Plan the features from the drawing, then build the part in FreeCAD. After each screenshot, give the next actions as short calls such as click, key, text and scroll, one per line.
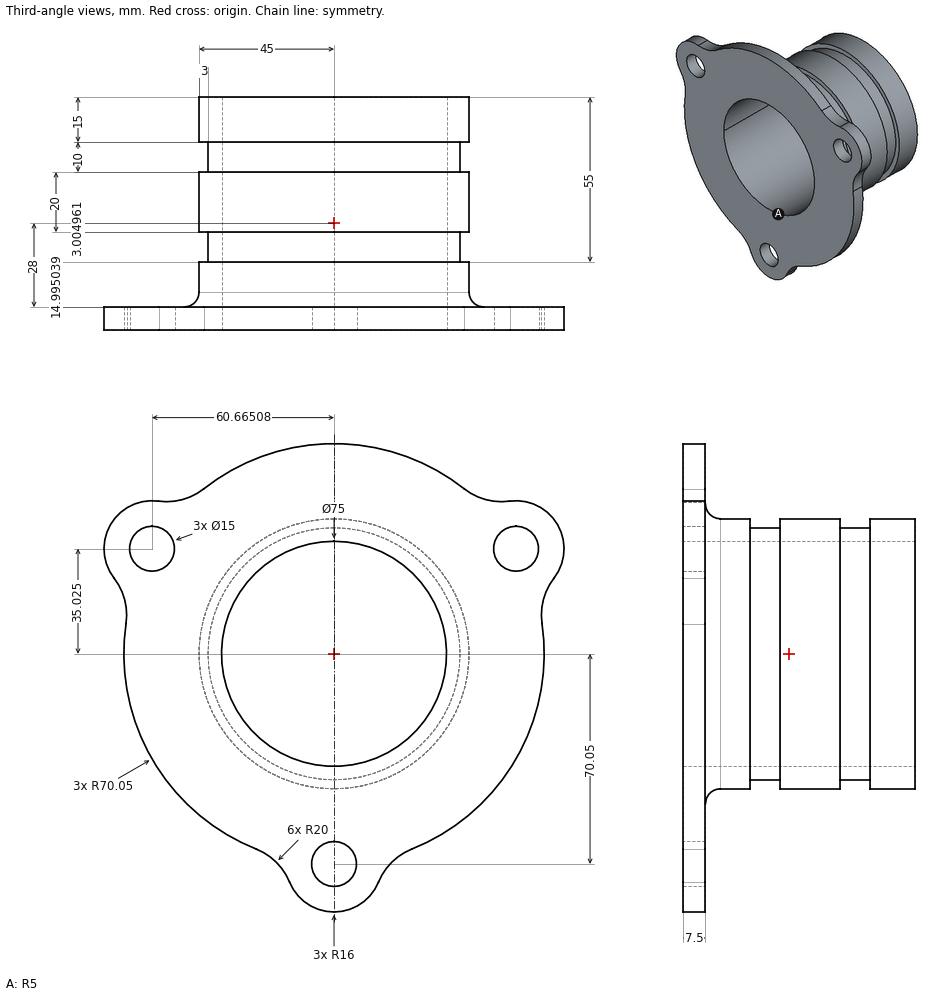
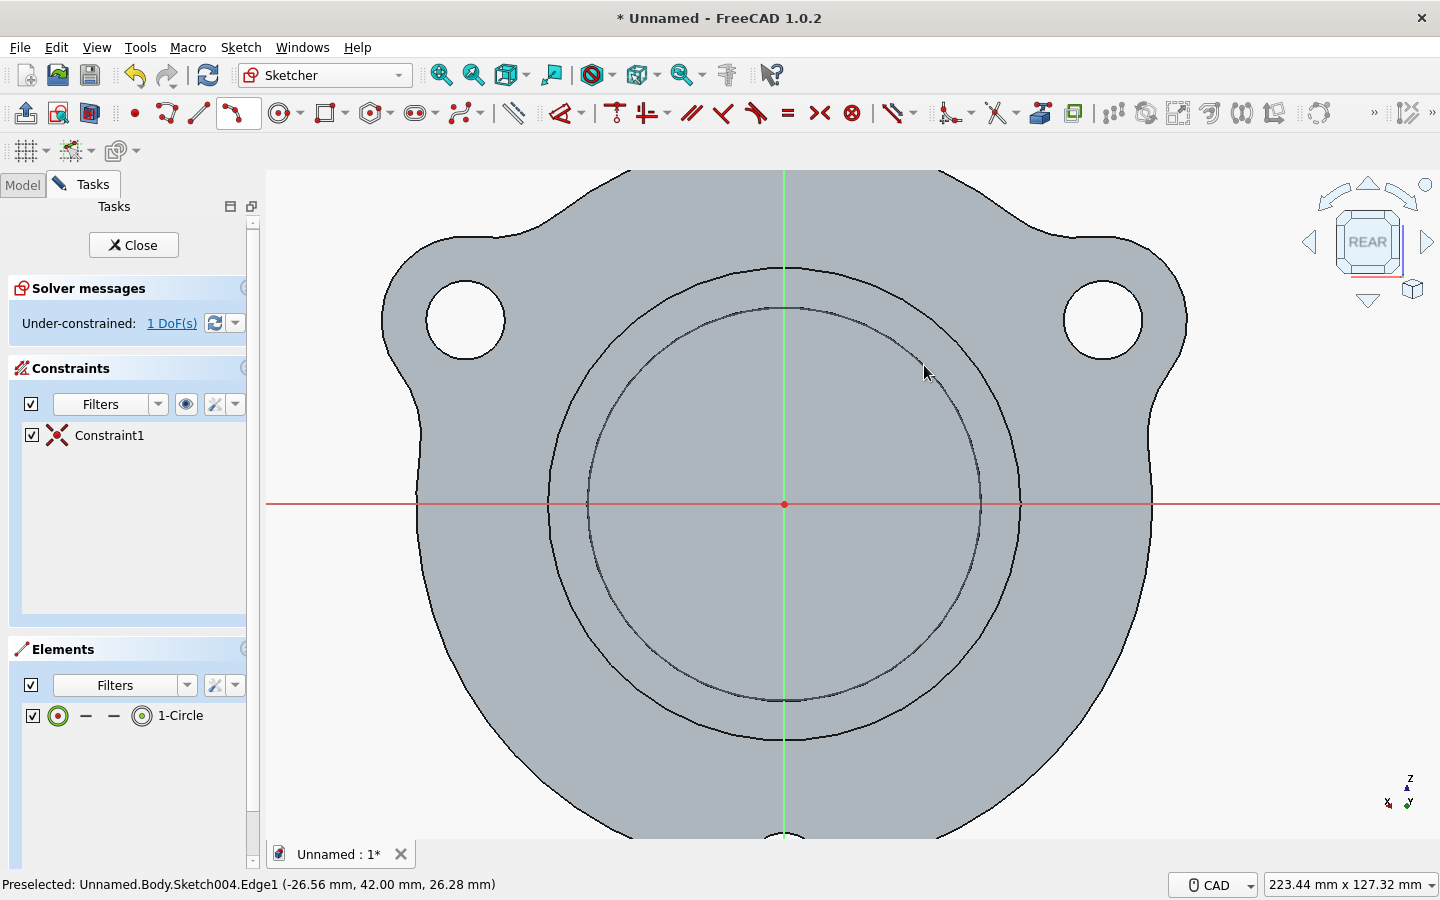
click(560, 114)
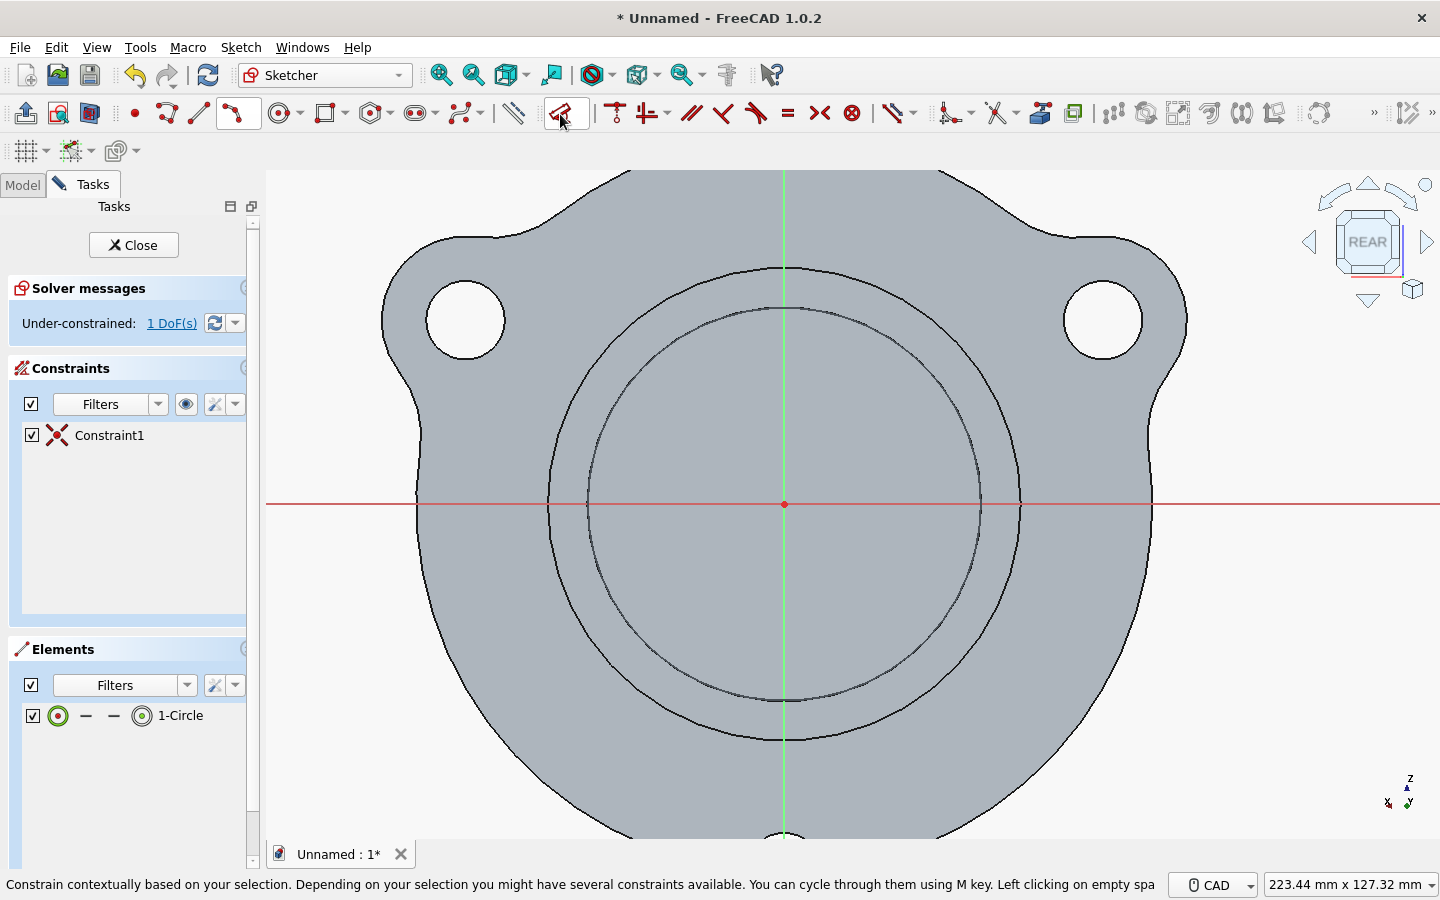
click(923, 365)
click(946, 342)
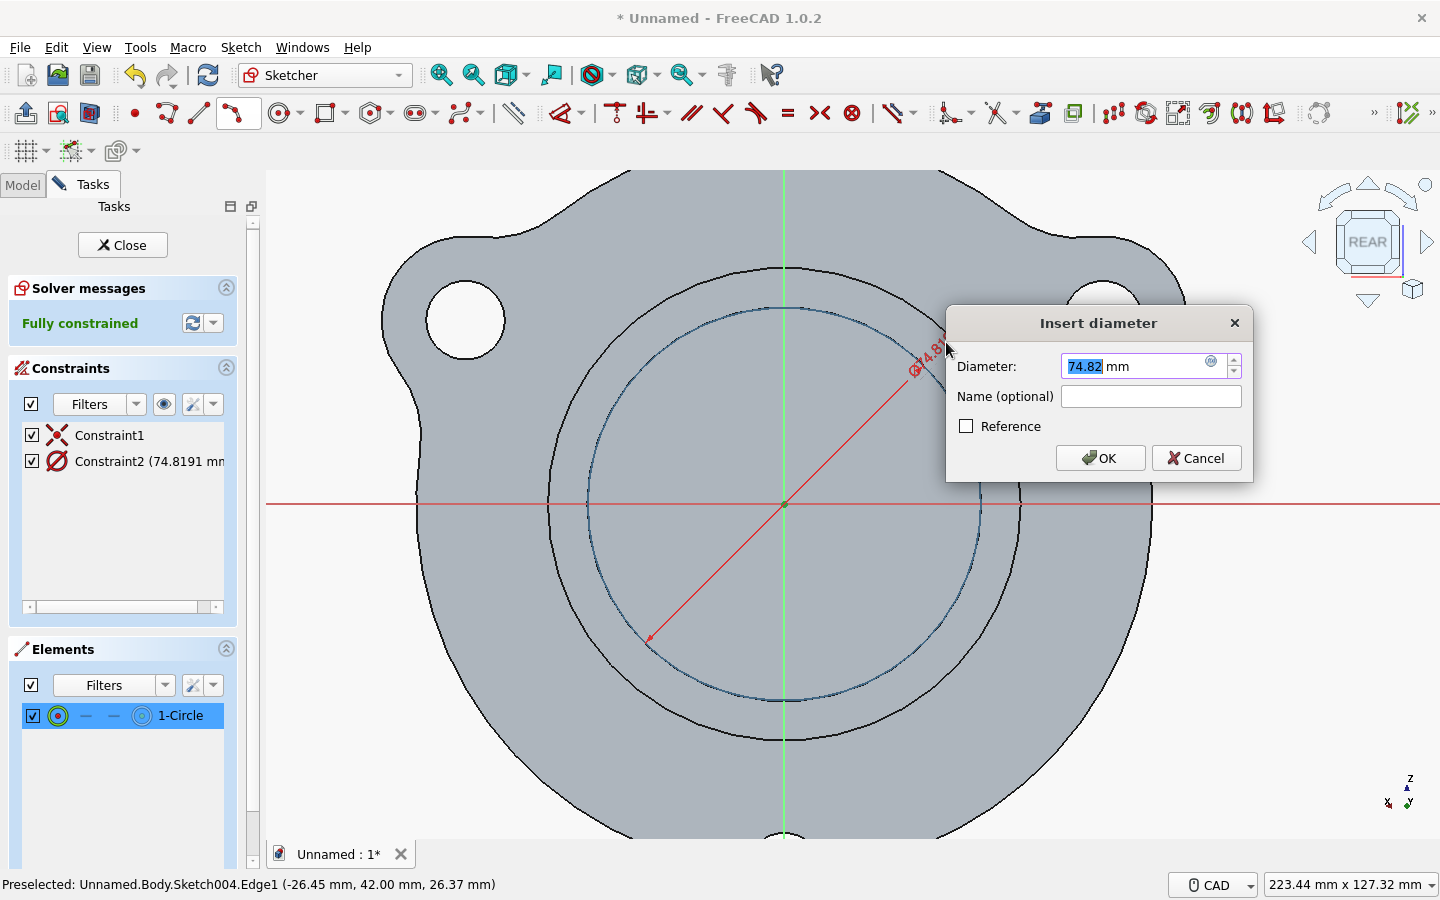
text(75)
key(Return)
key(Escape)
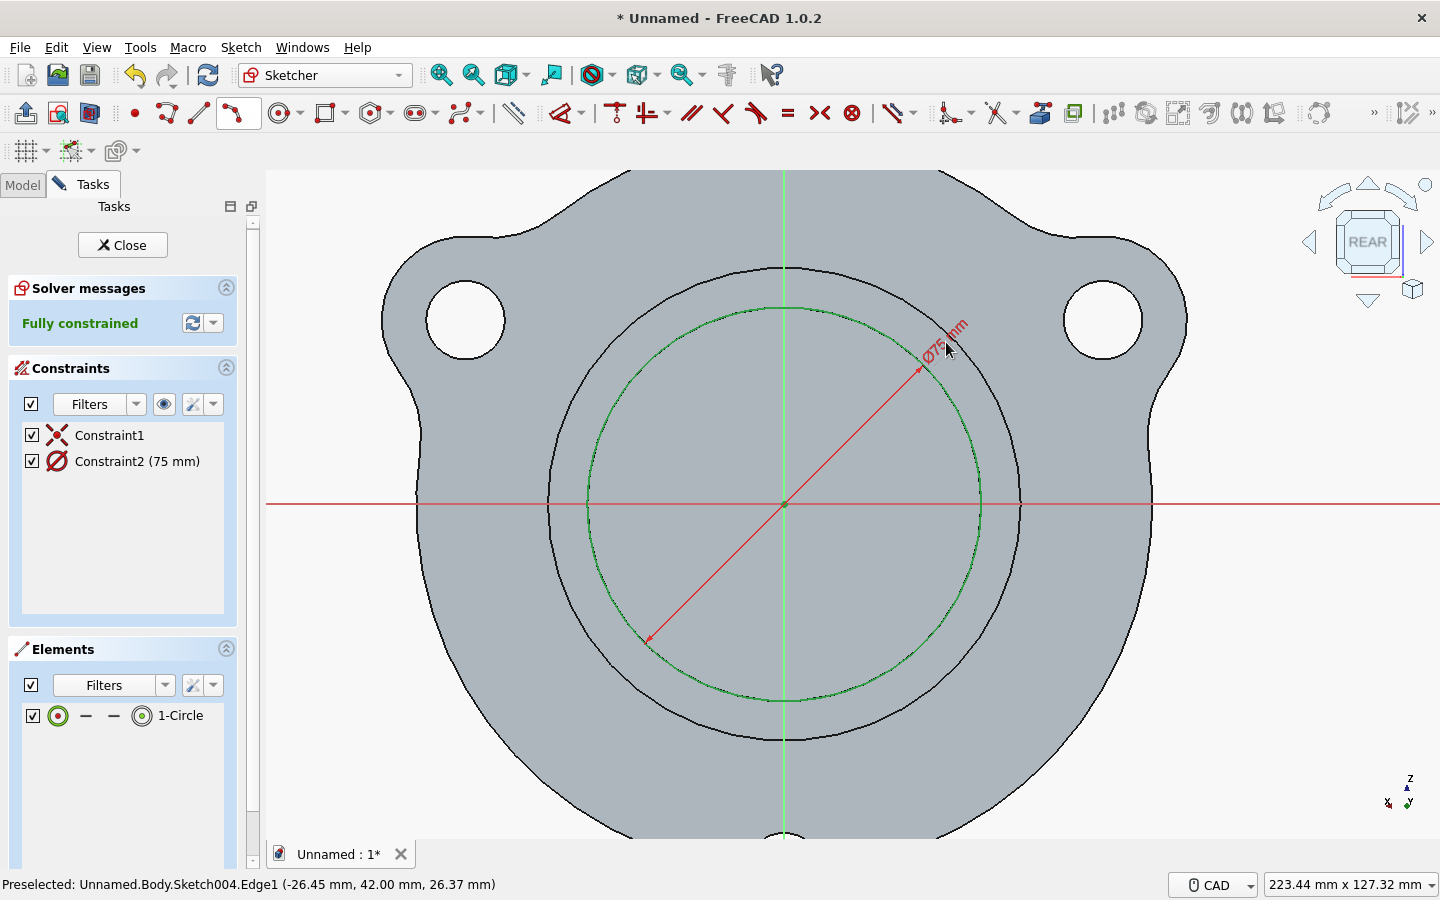
click(123, 245)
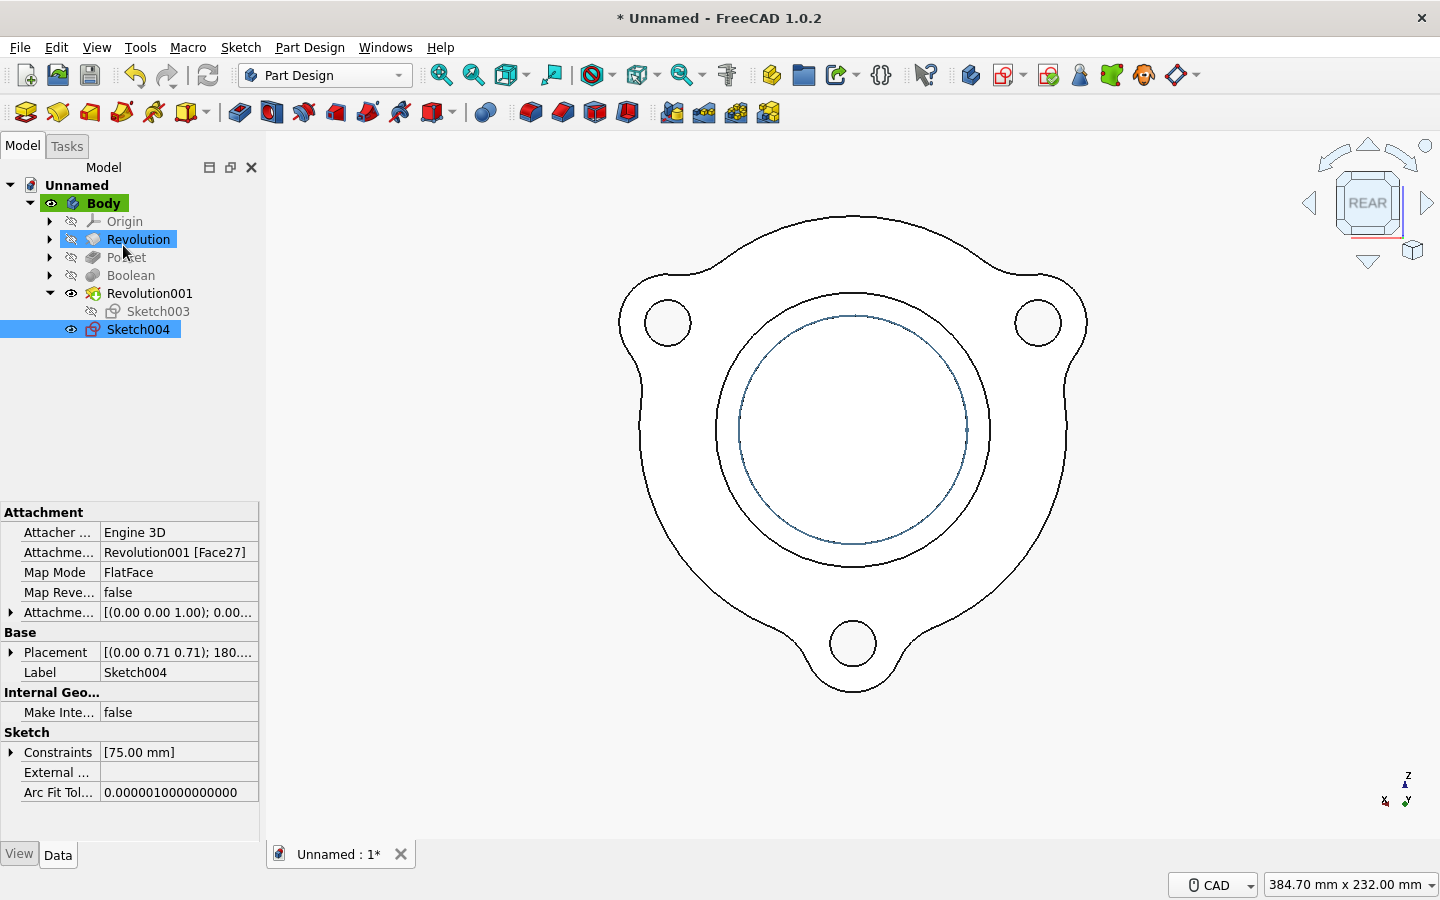
click(240, 112)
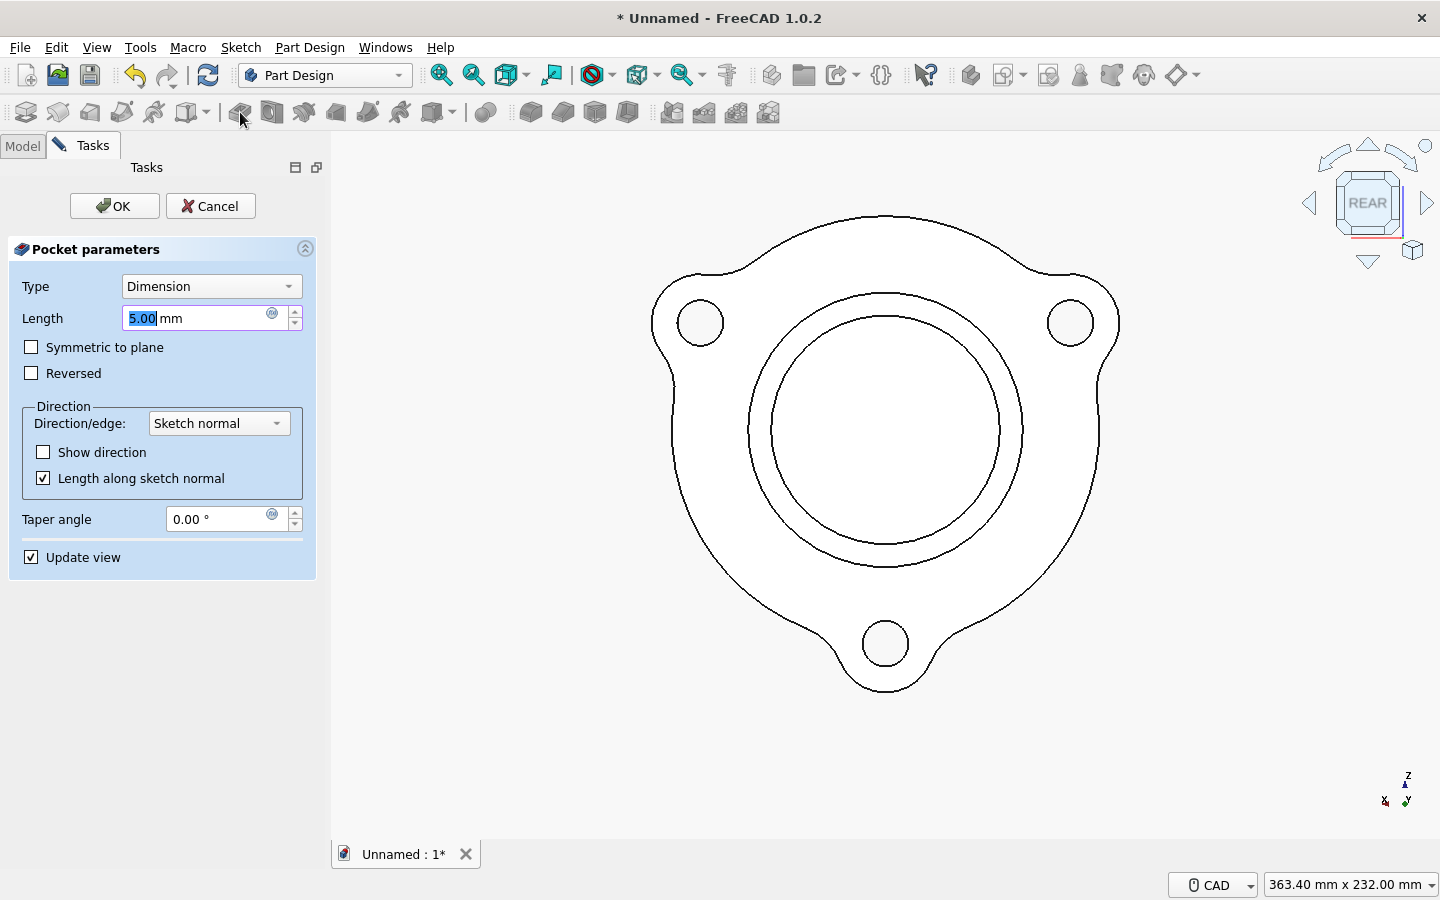
click(212, 286)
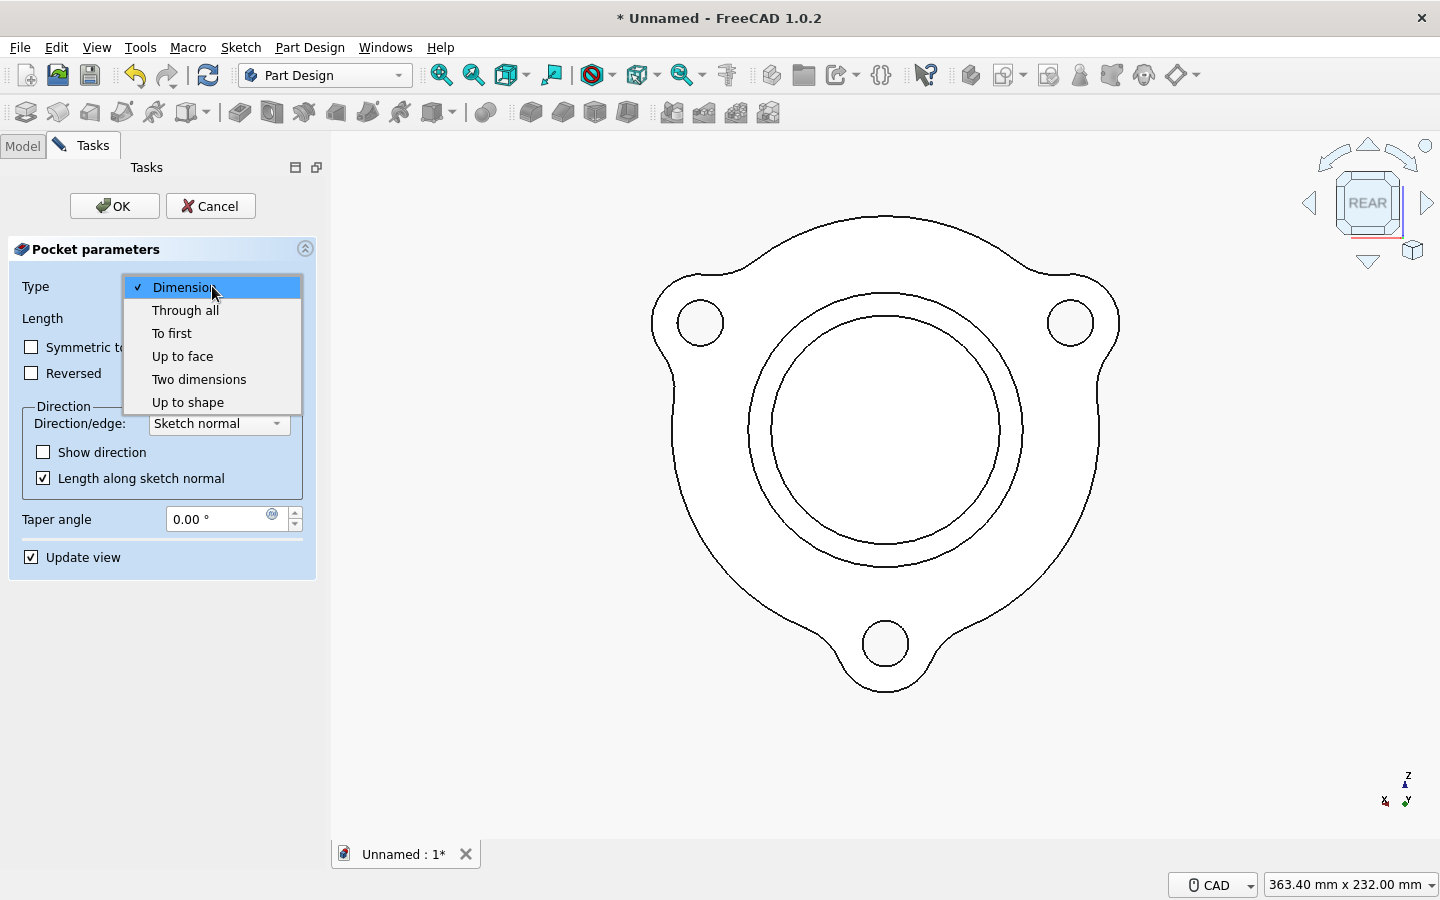
click(212, 310)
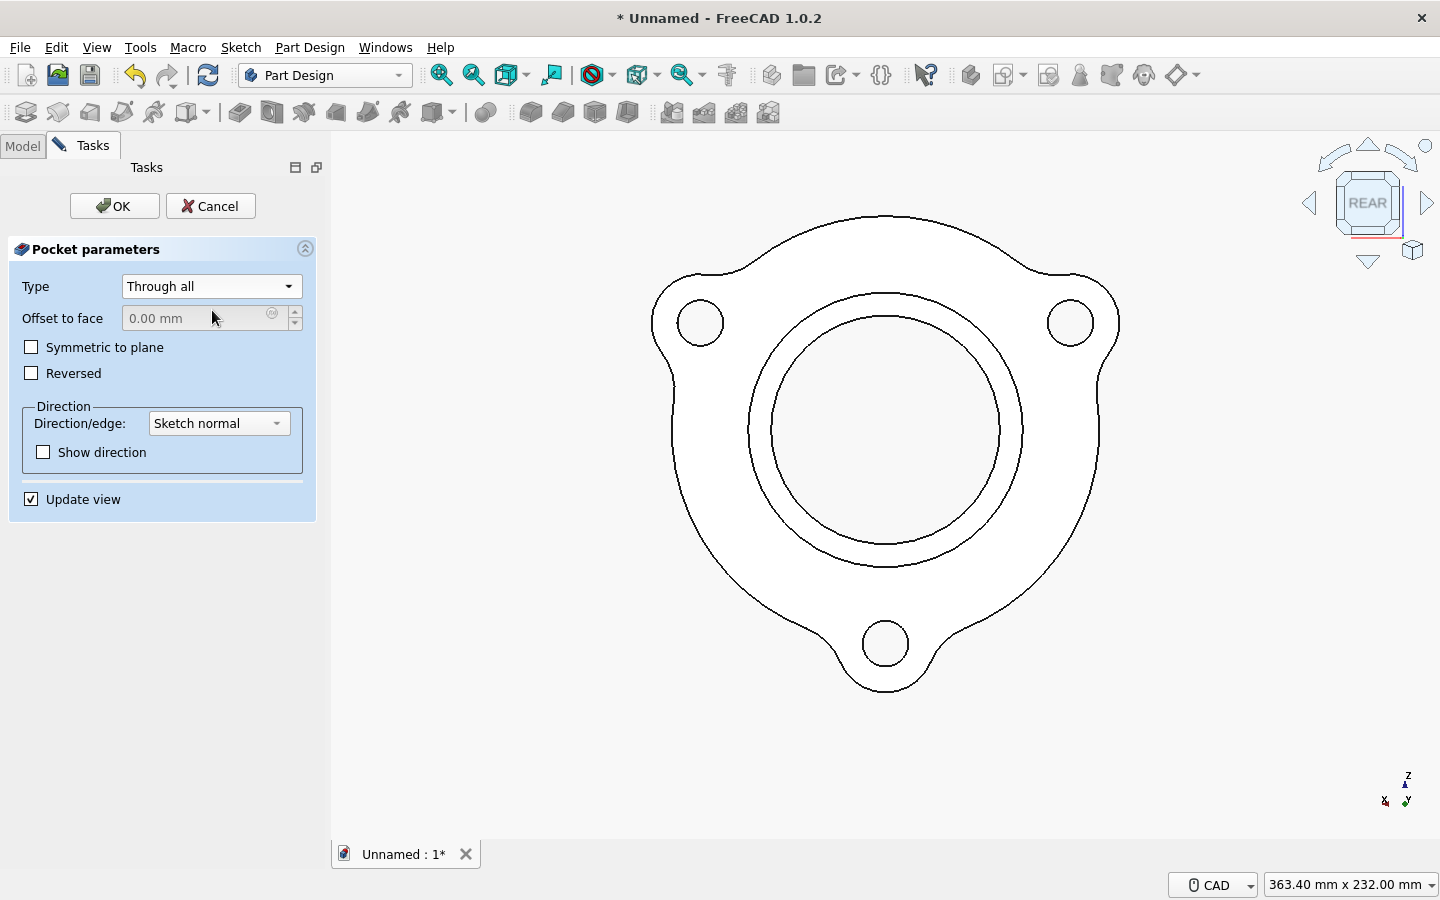
click(115, 206)